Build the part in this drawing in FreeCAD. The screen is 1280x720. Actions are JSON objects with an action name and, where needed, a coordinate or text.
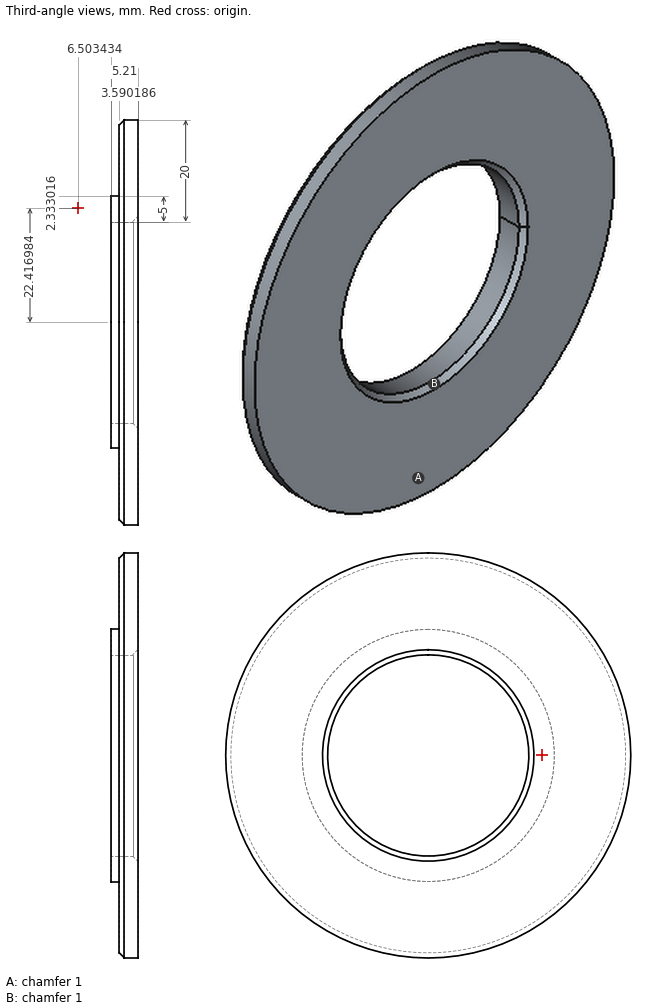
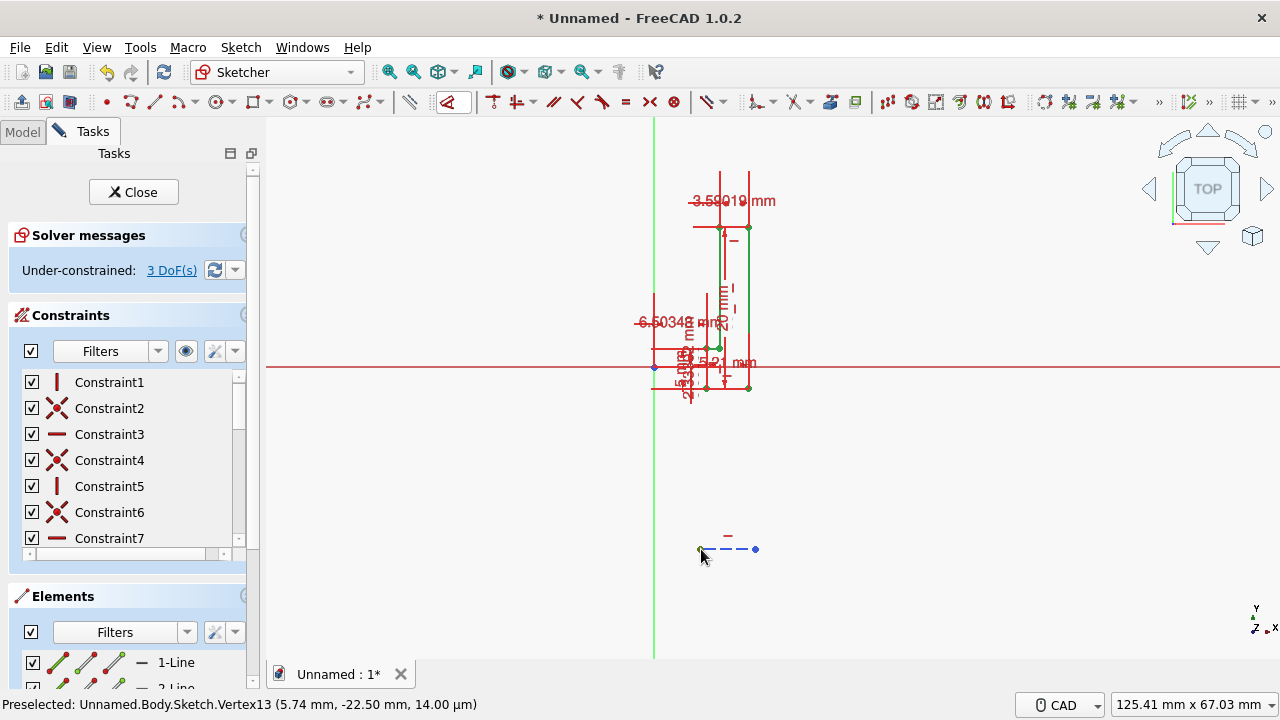
{"action": "key", "text": "i"}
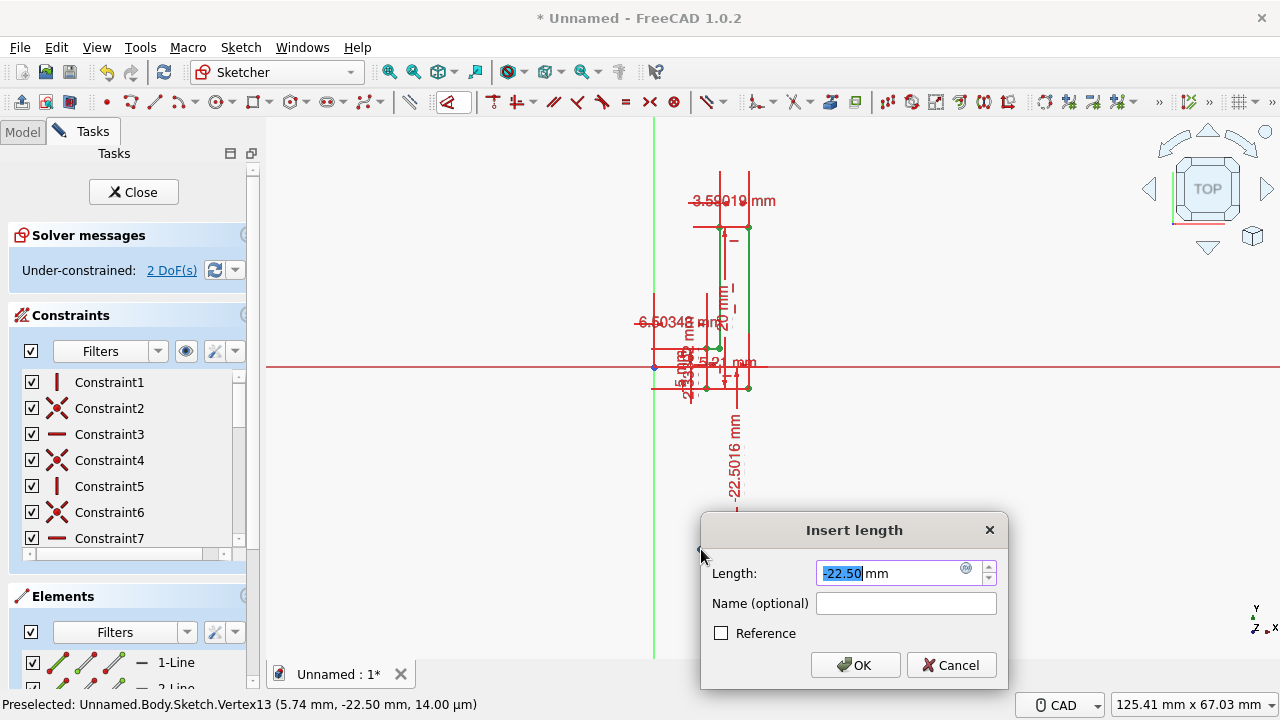
{"action": "type", "text": "-22.416984"}
{"action": "key", "text": "Return"}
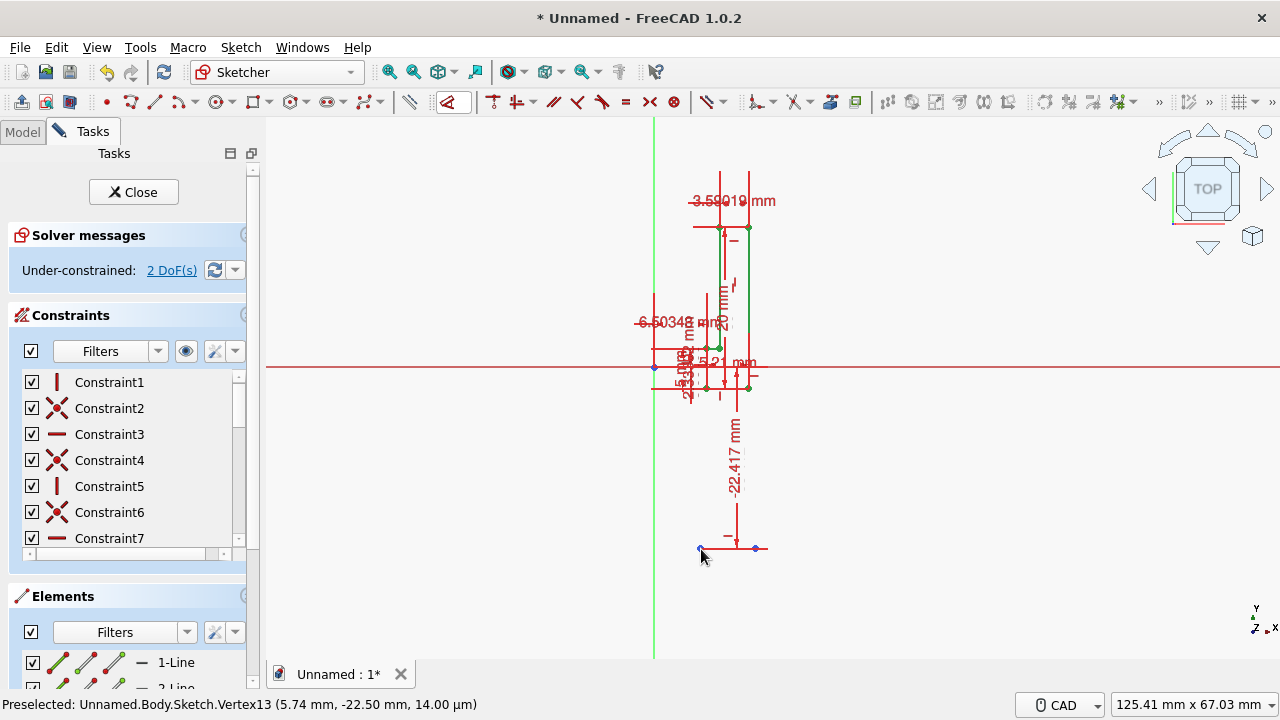
{"action": "left_click", "coordinate": [134, 192]}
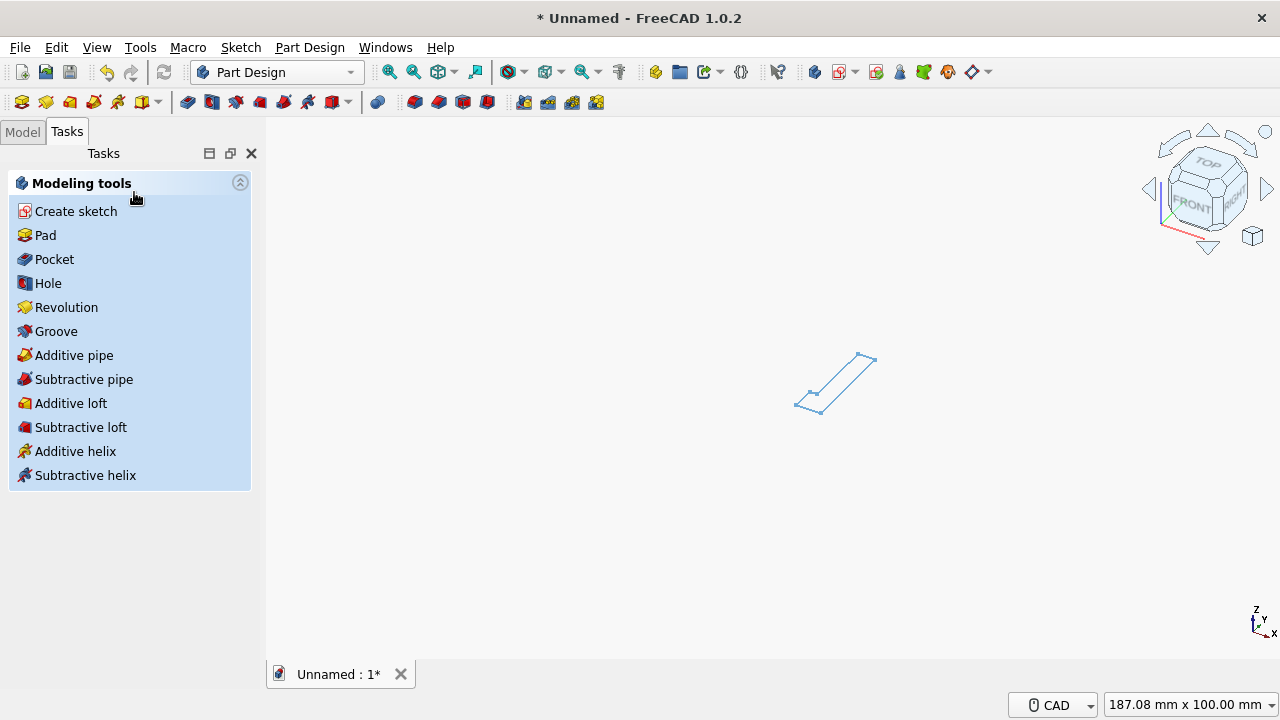
{"action": "left_click", "coordinate": [46, 102]}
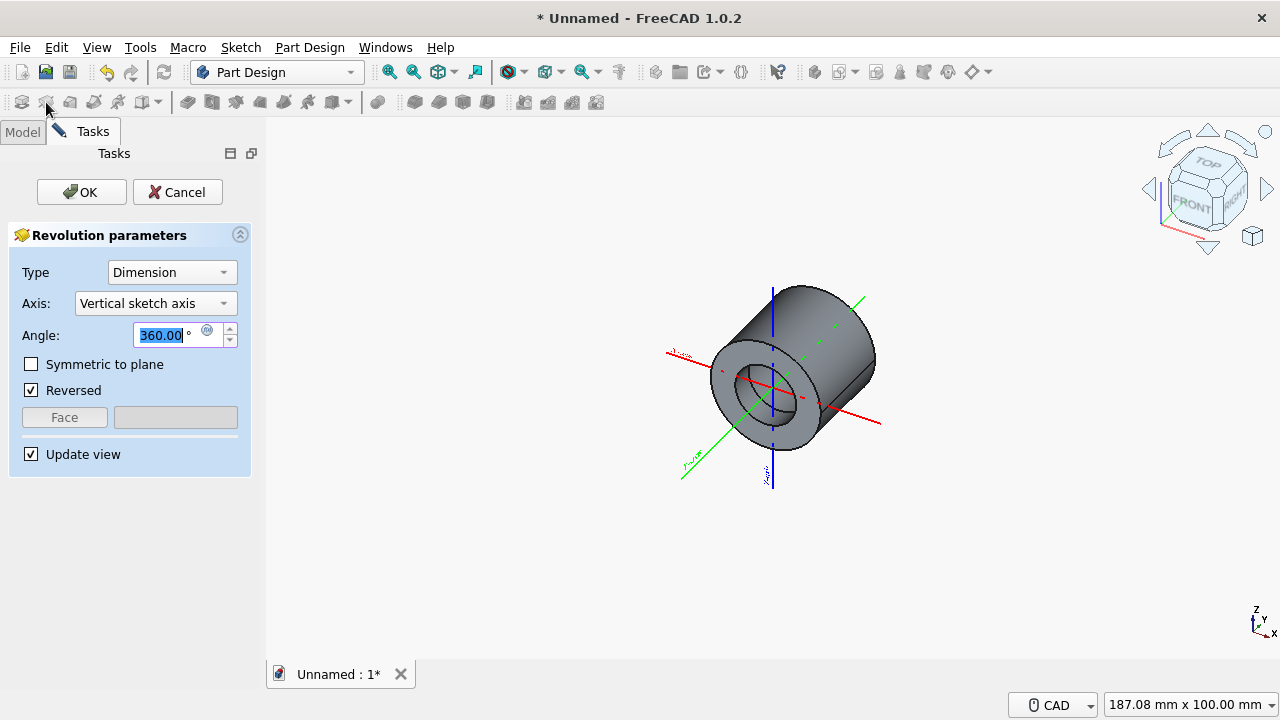
{"action": "left_click", "coordinate": [156, 304]}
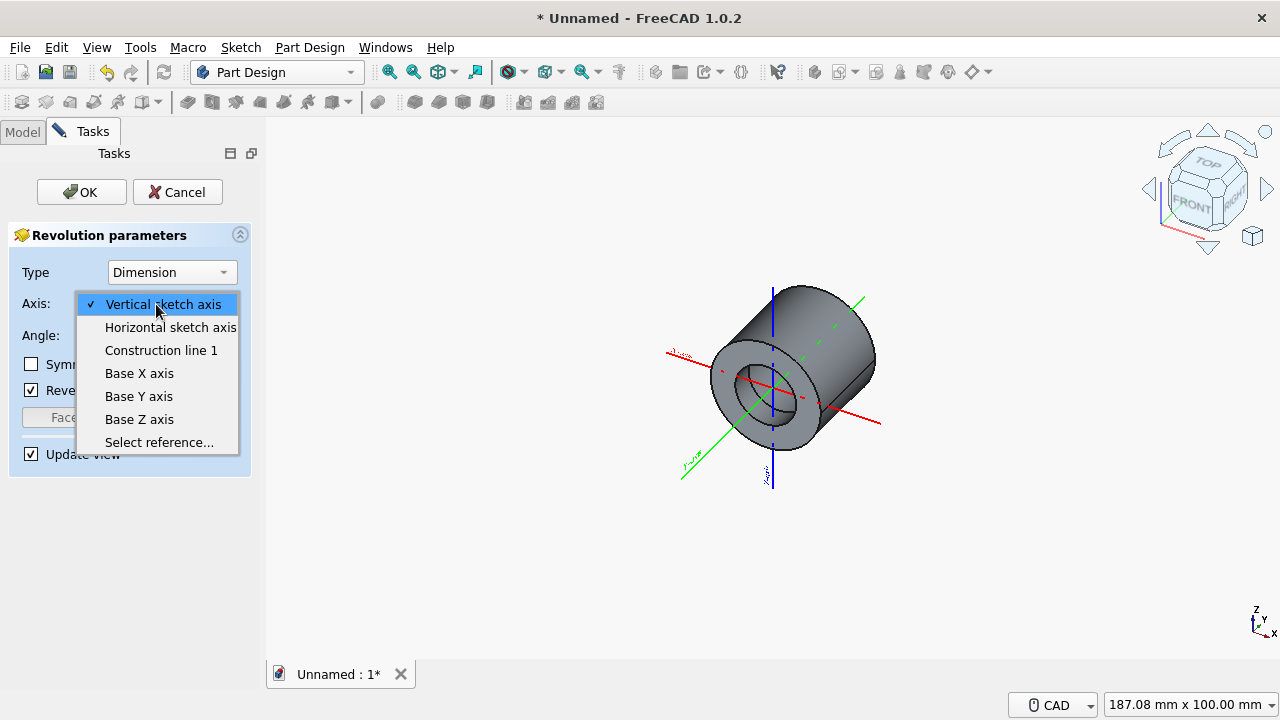
{"action": "left_click", "coordinate": [156, 350]}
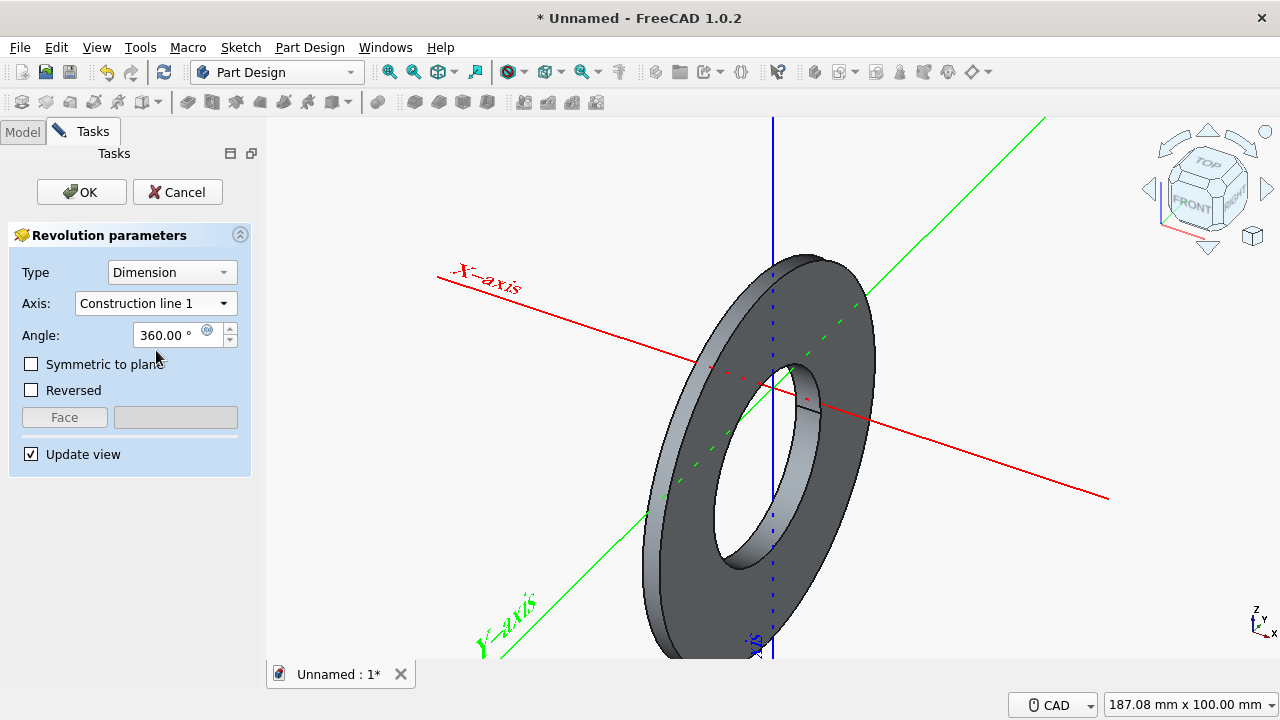
{"action": "left_click", "coordinate": [82, 192]}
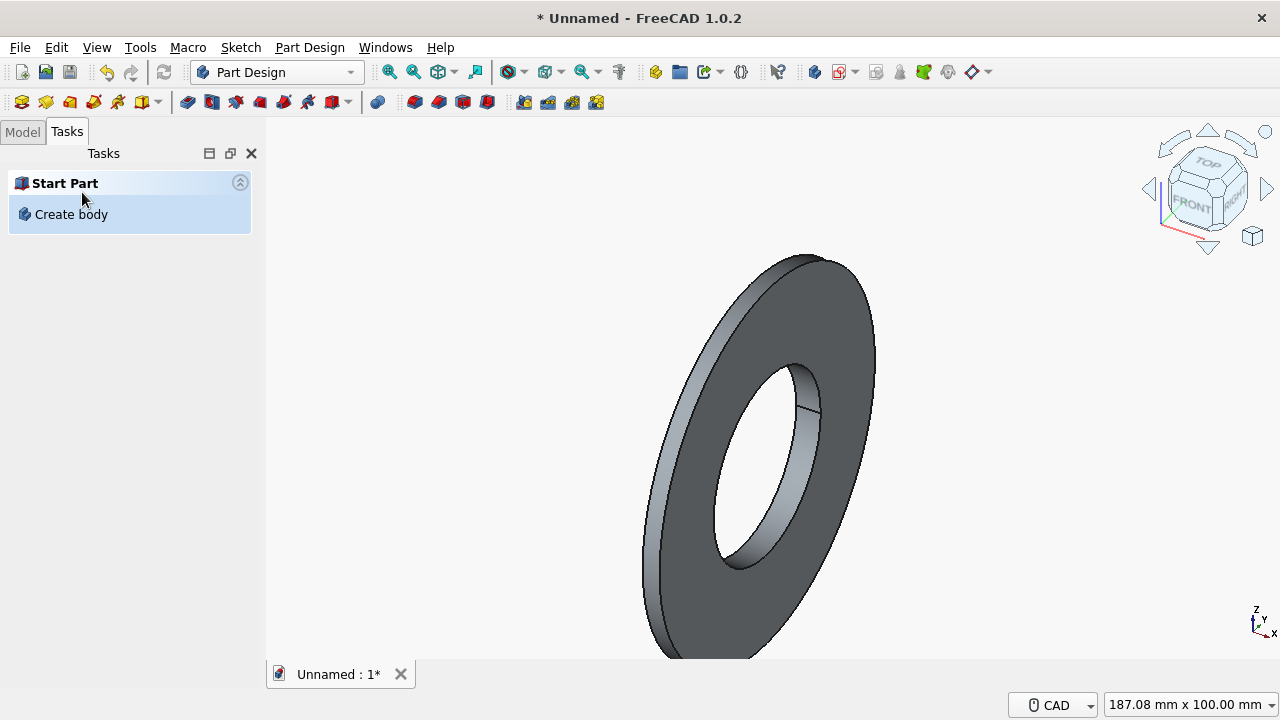
{"action": "key", "text": "v f"}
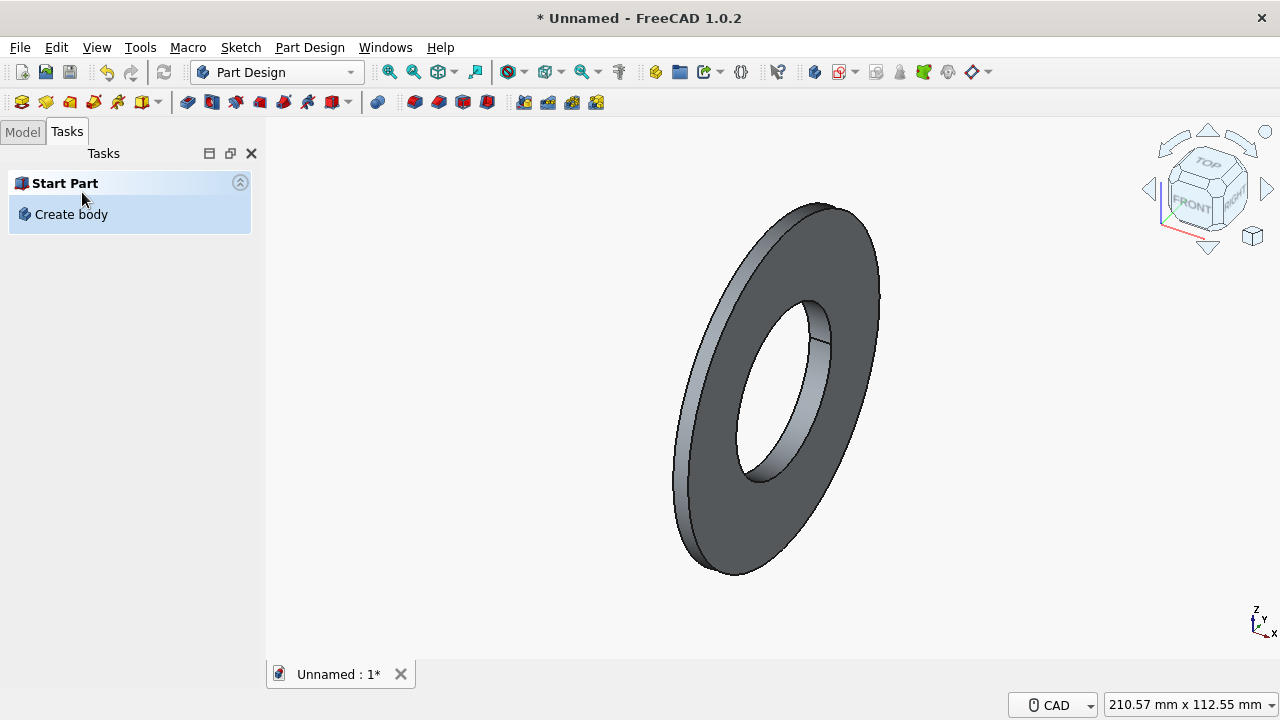
{"action": "key", "text": "0"}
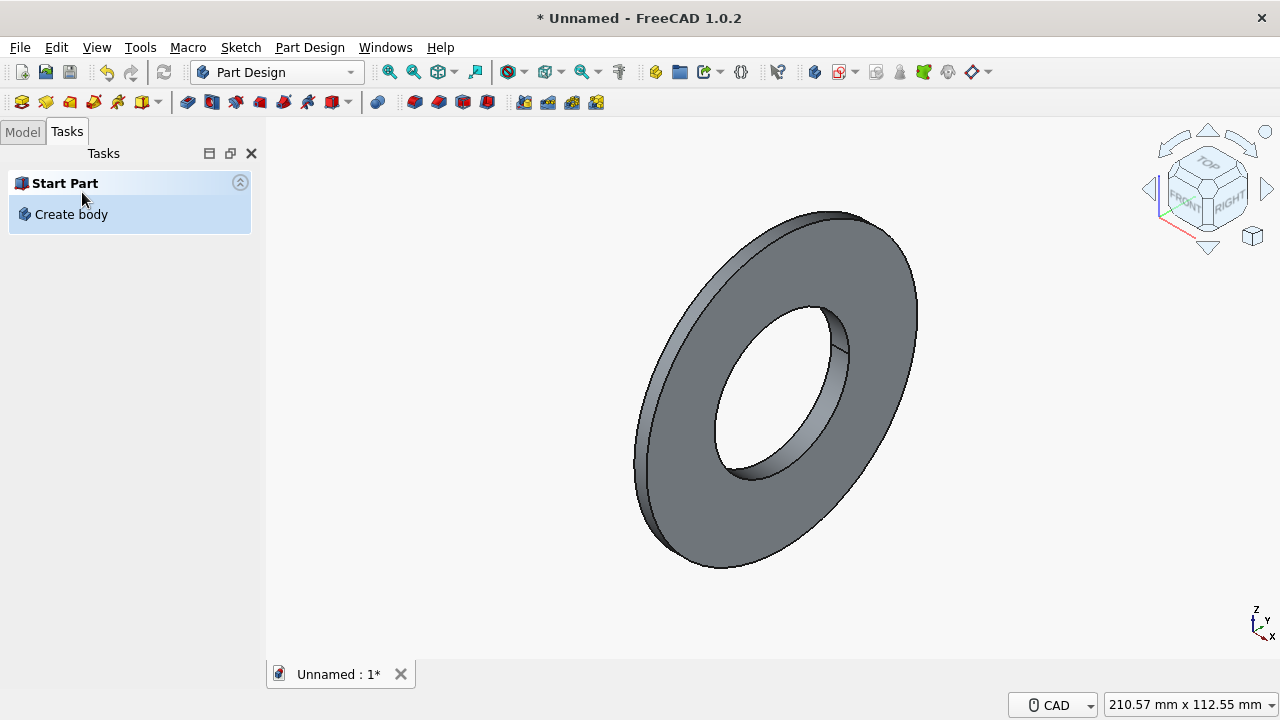
{"action": "key", "text": "2"}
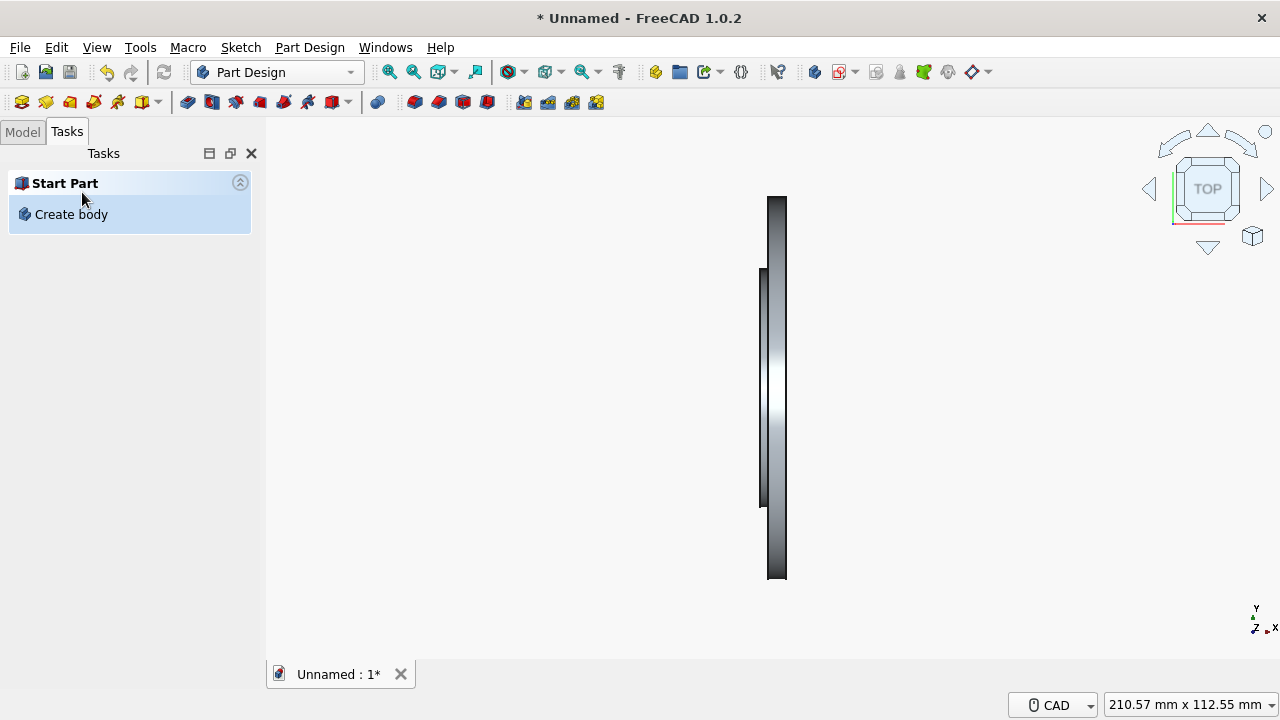
{"action": "left_click", "coordinate": [768, 542]}